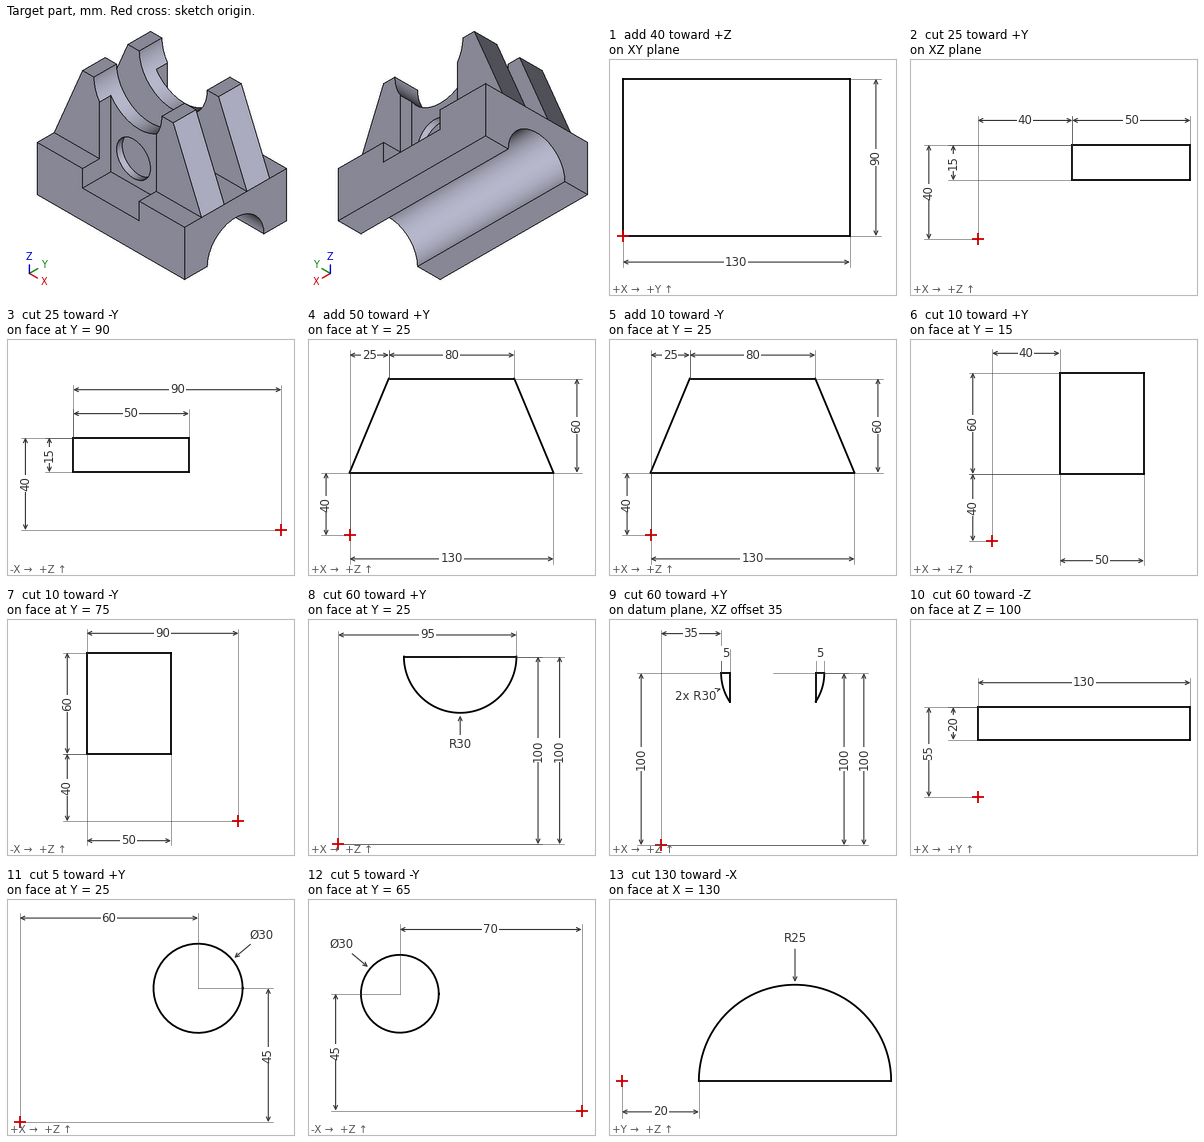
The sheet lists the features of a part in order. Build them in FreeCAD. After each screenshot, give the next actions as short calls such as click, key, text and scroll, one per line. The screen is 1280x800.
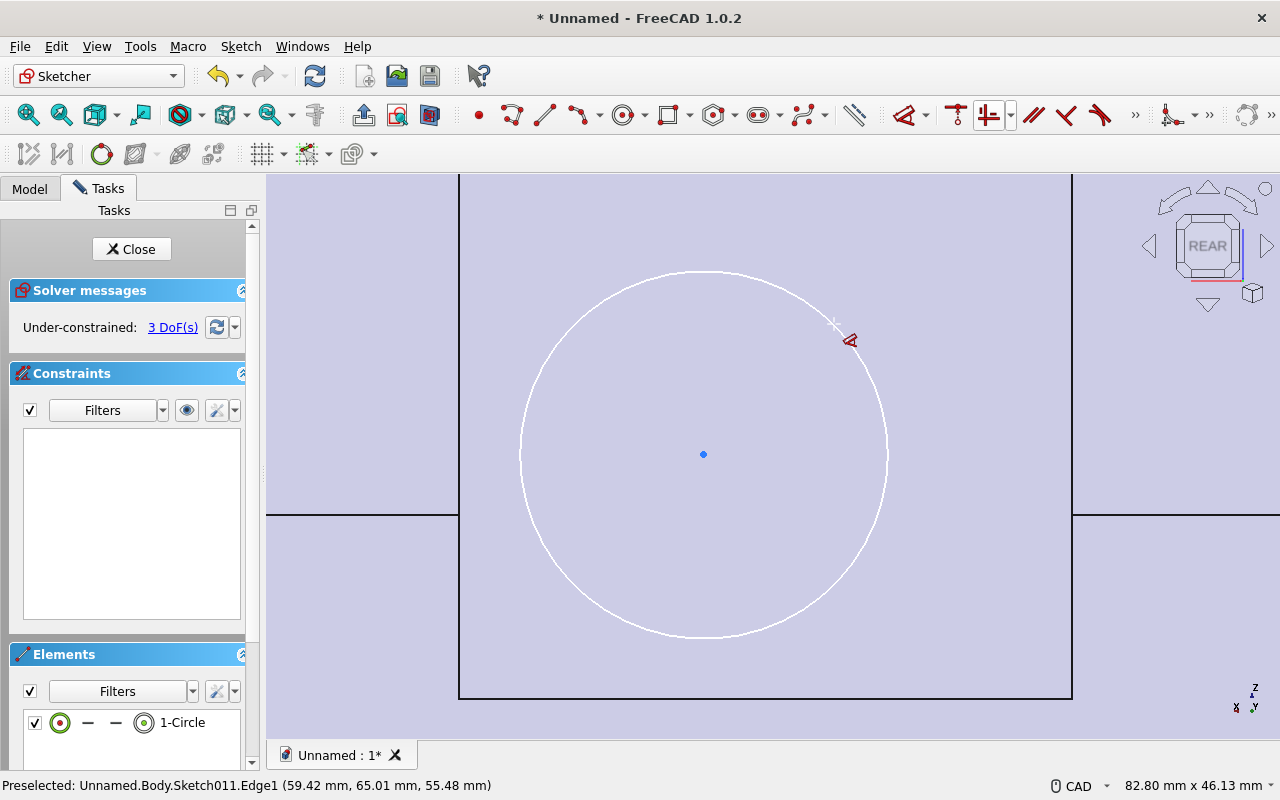
click(834, 325)
click(857, 302)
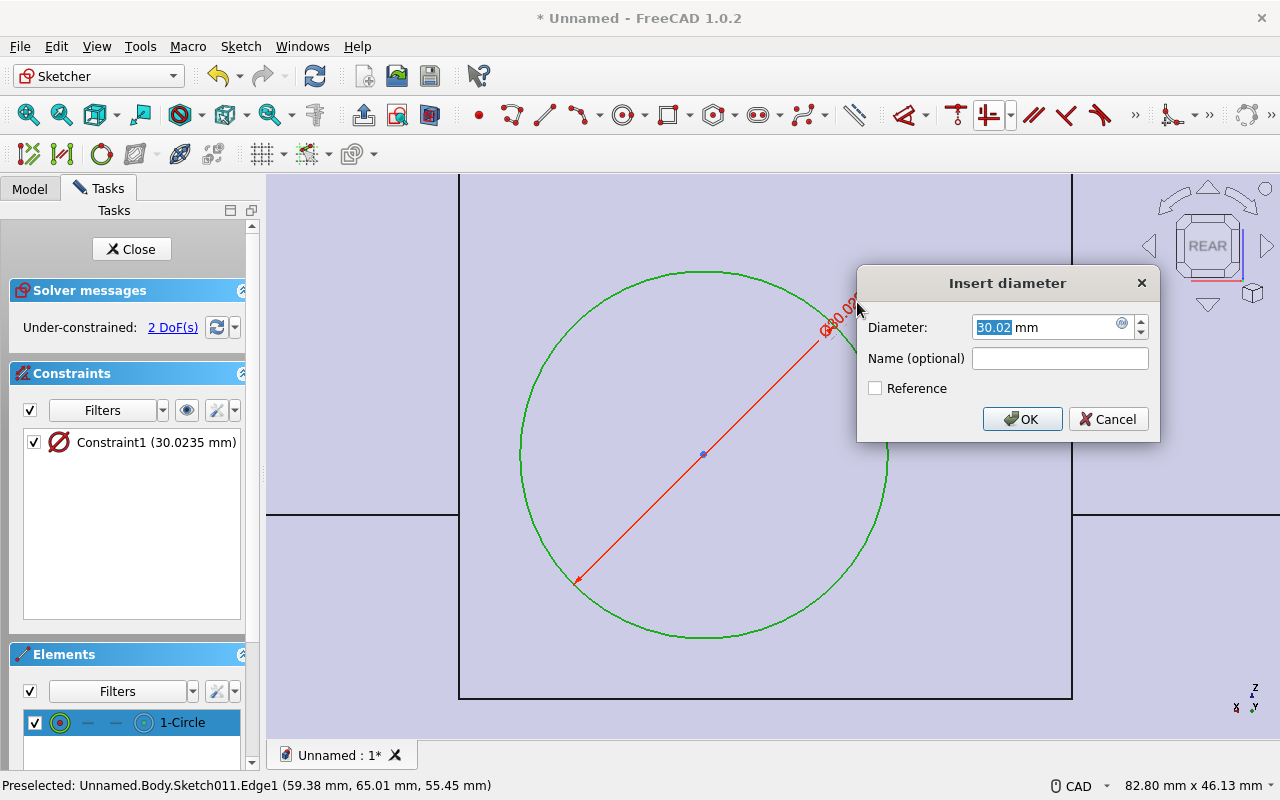
text(30)
key(Return)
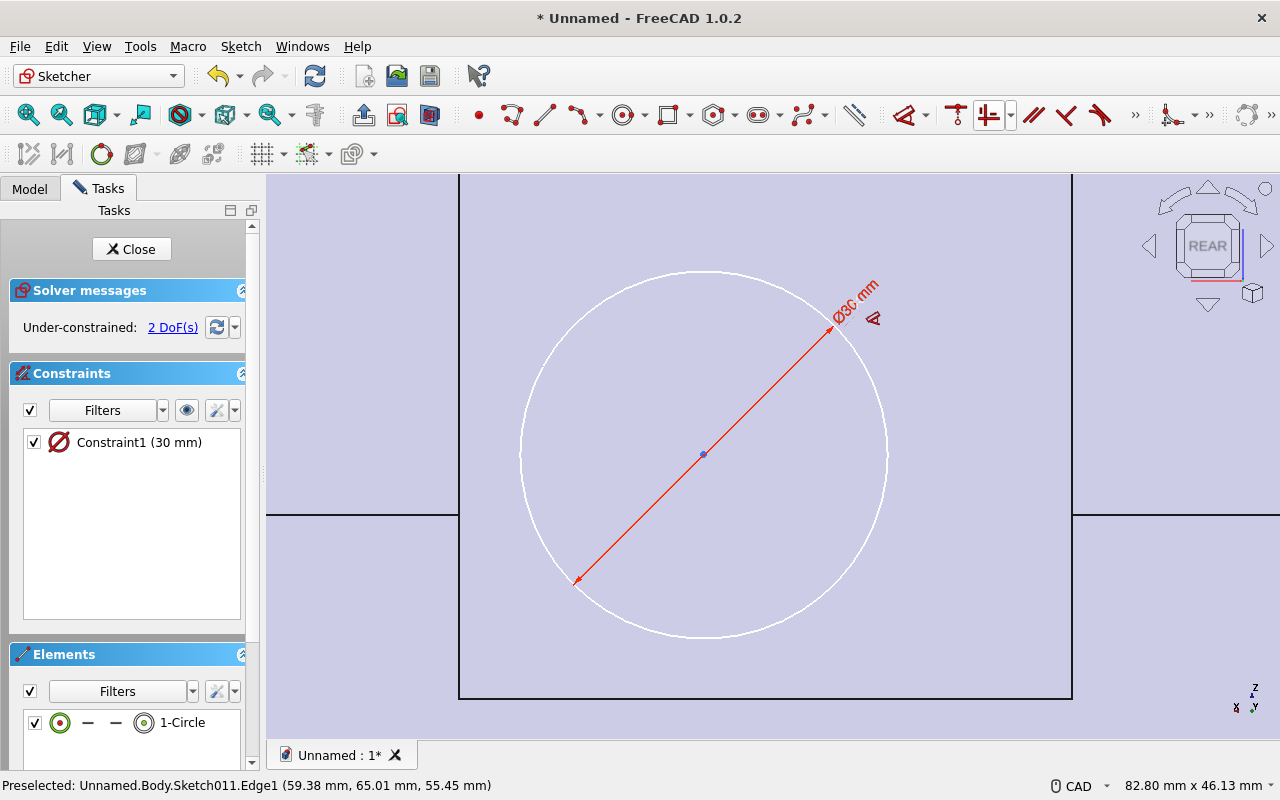
click(704, 455)
click(910, 421)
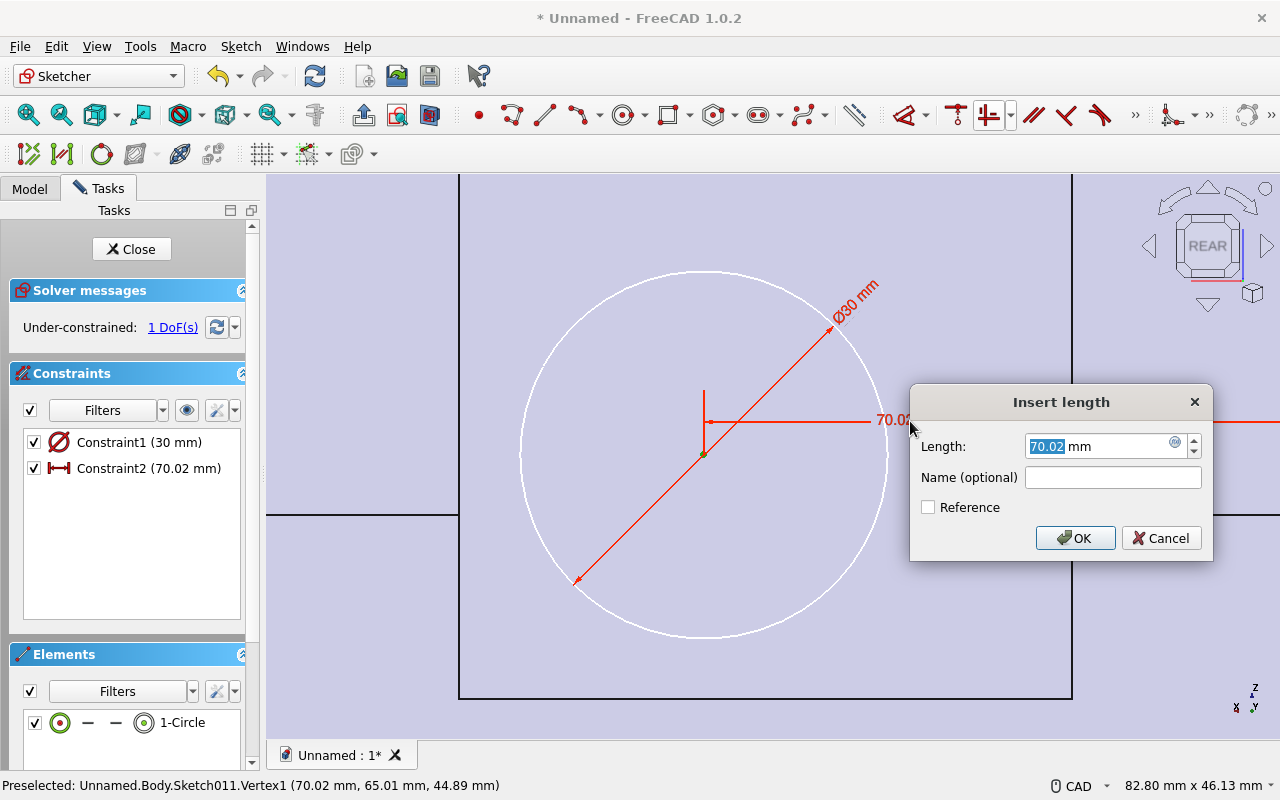
text(70)
key(Return)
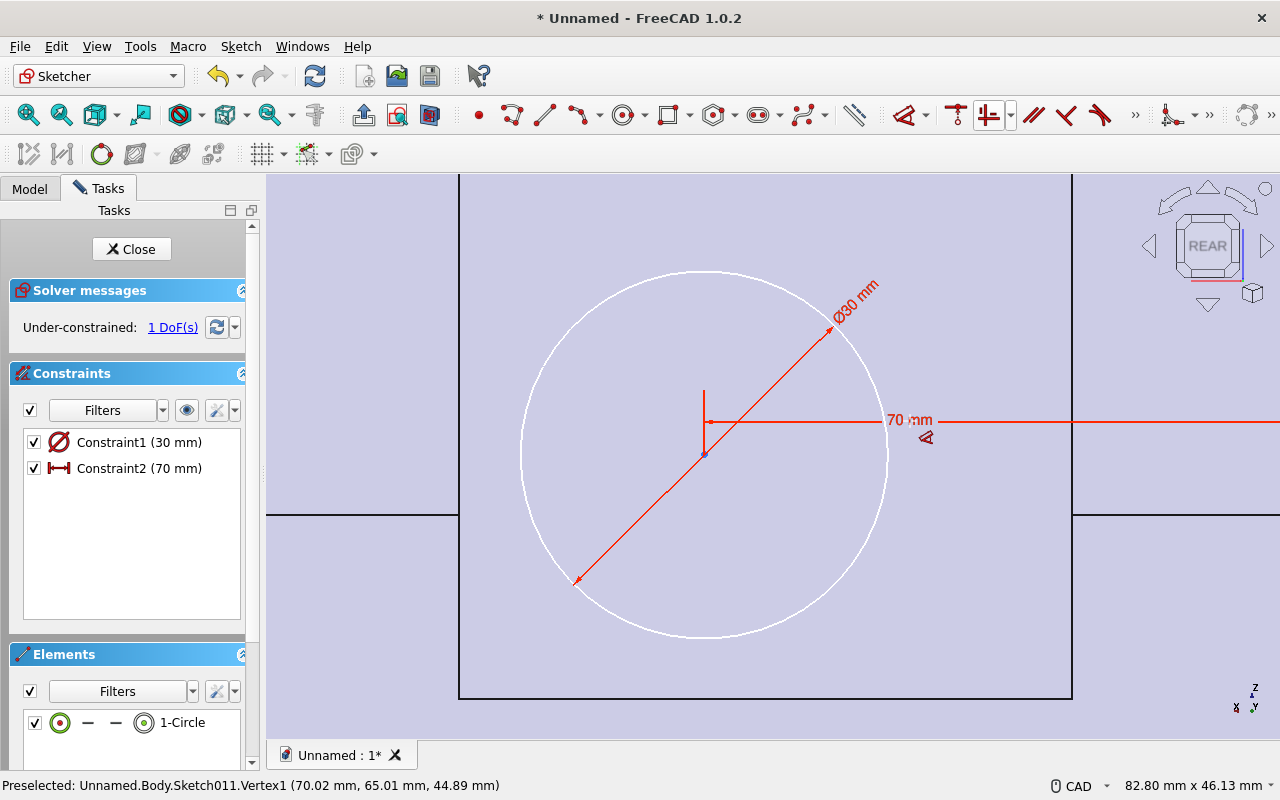
click(704, 455)
click(670, 583)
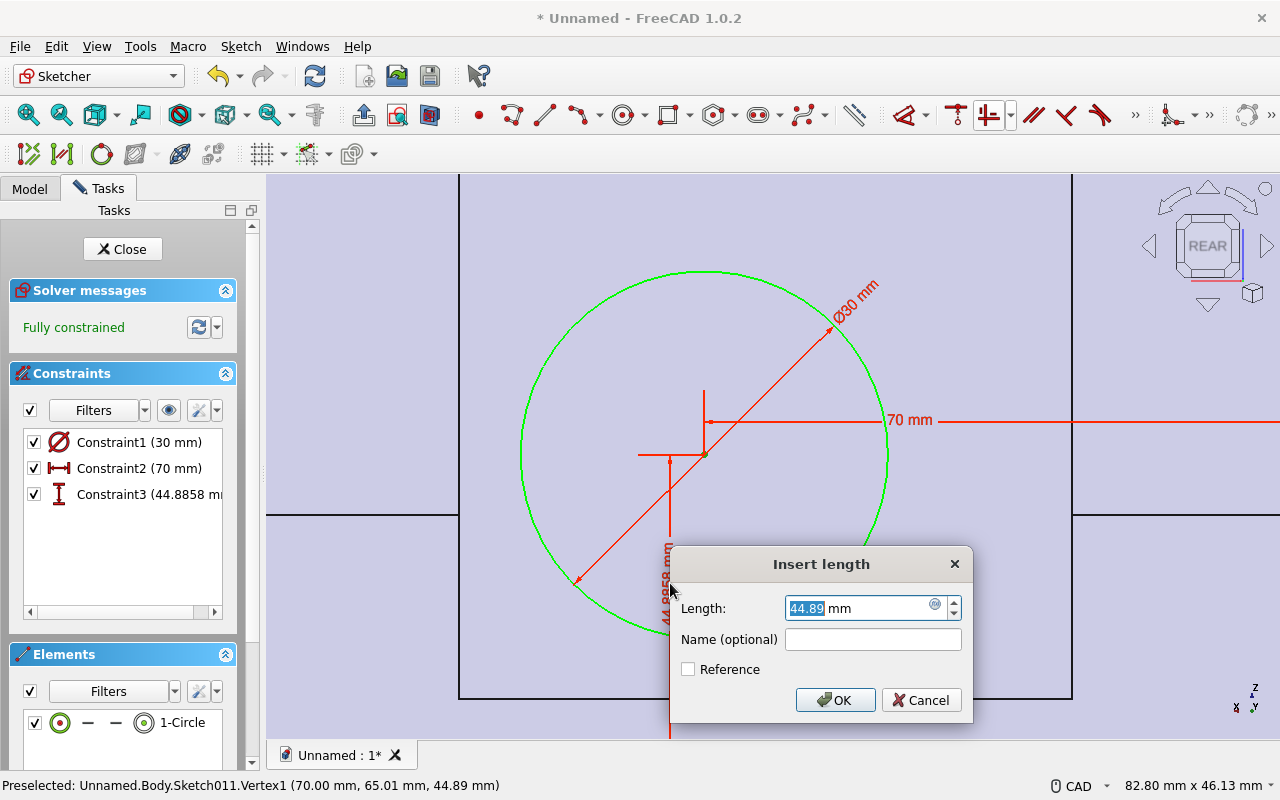
text(45)
key(Return)
key(Escape)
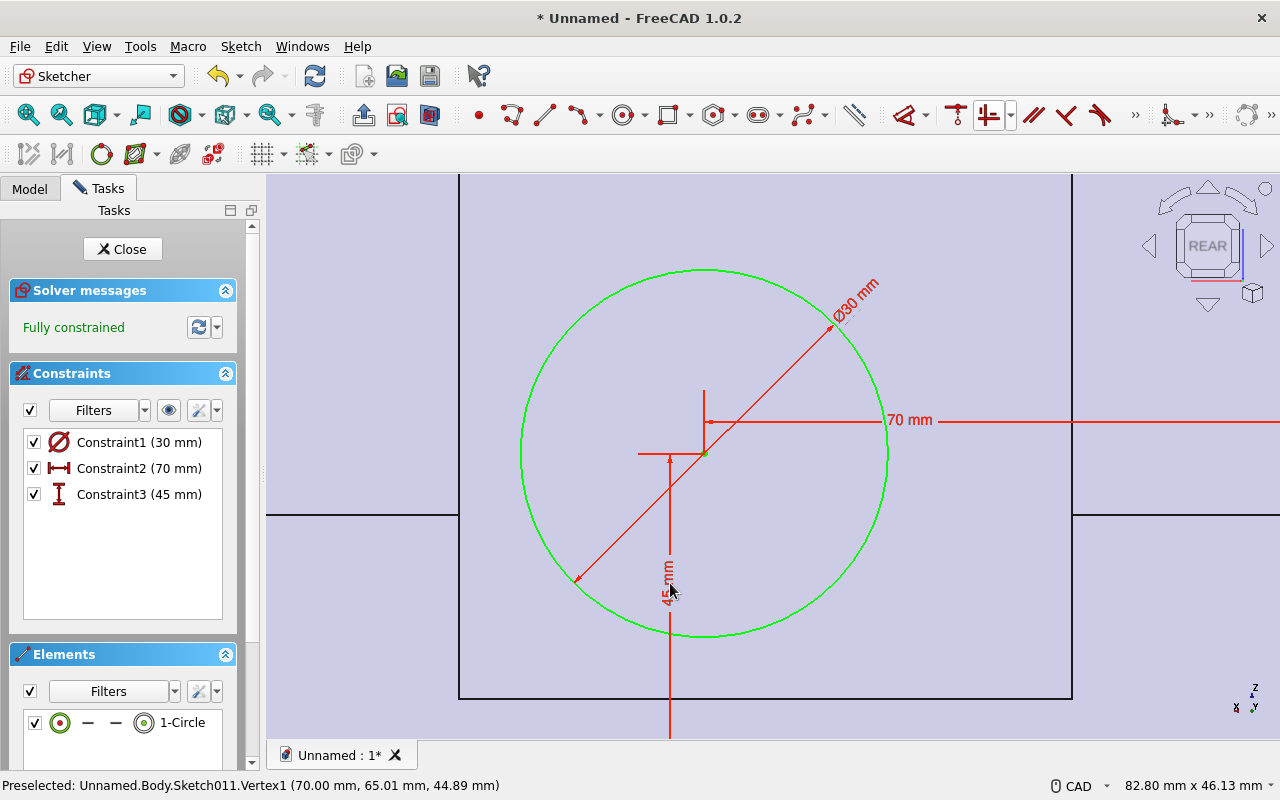
click(123, 249)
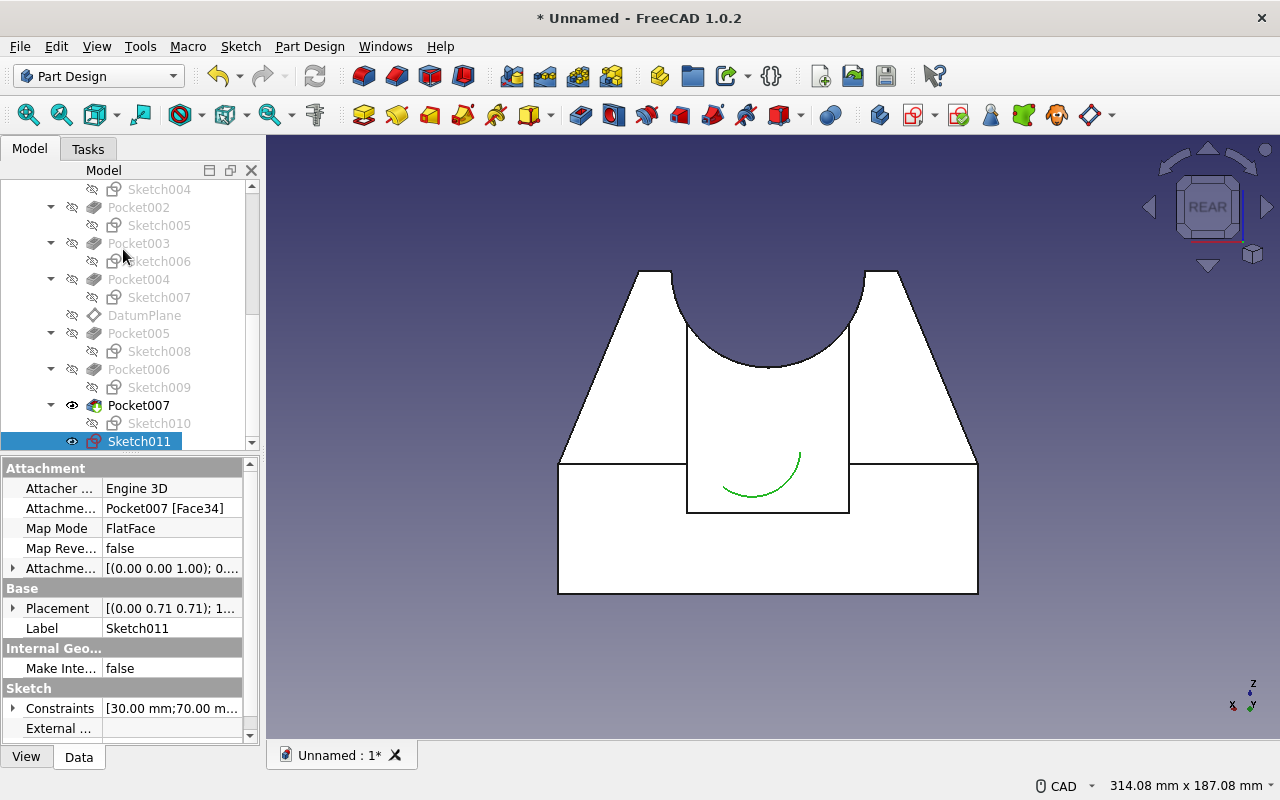
click(581, 116)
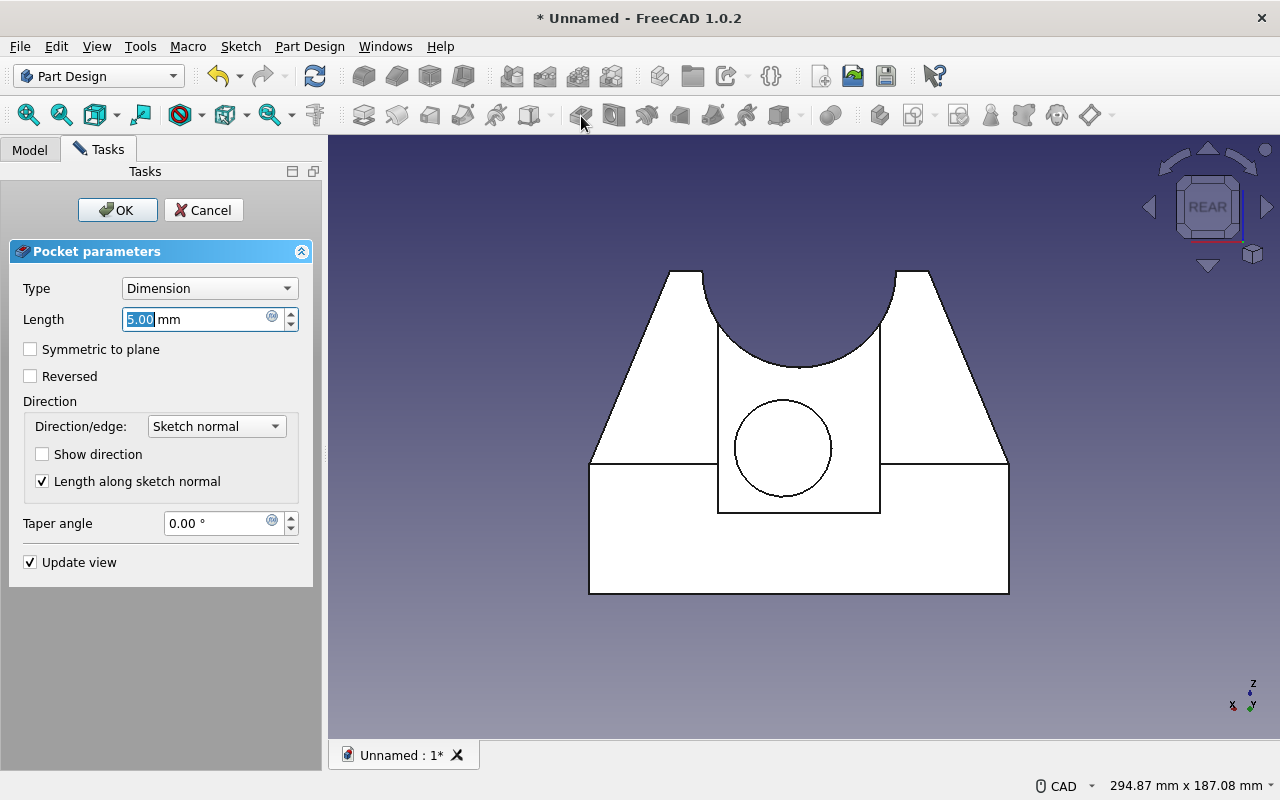
text(5)
key(Tab)